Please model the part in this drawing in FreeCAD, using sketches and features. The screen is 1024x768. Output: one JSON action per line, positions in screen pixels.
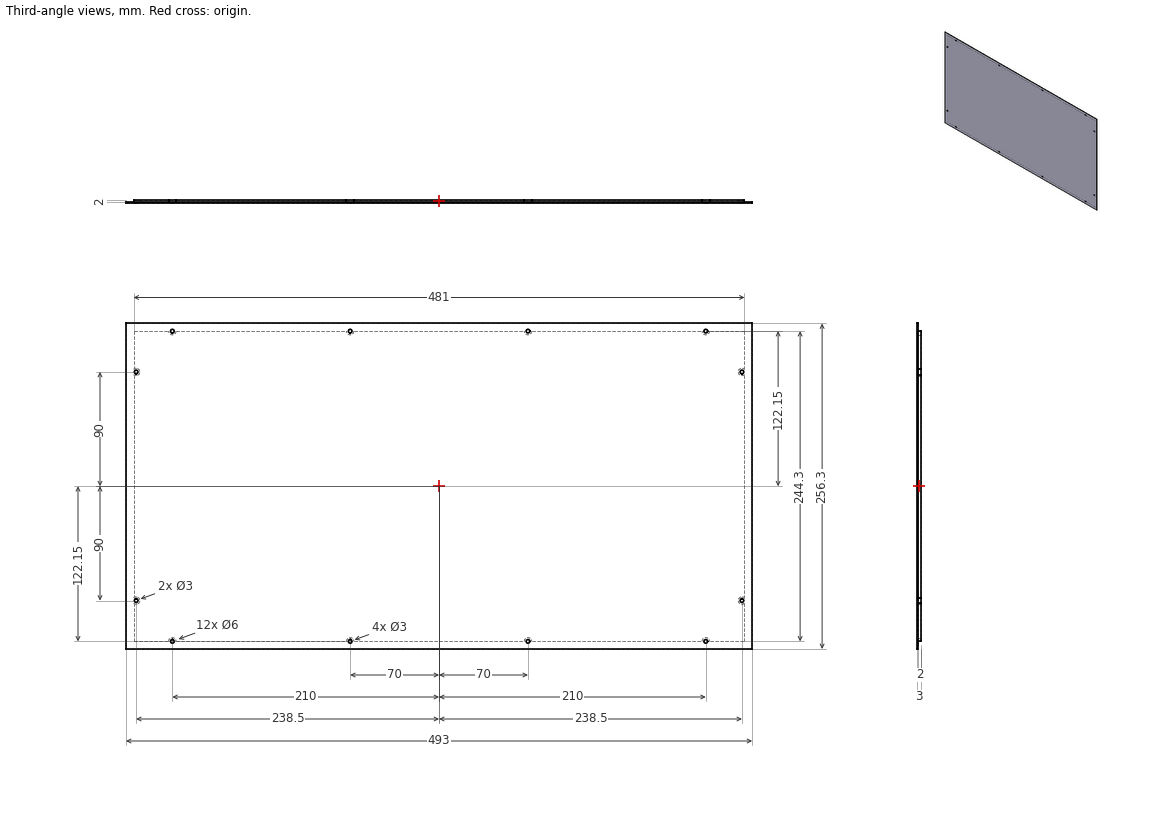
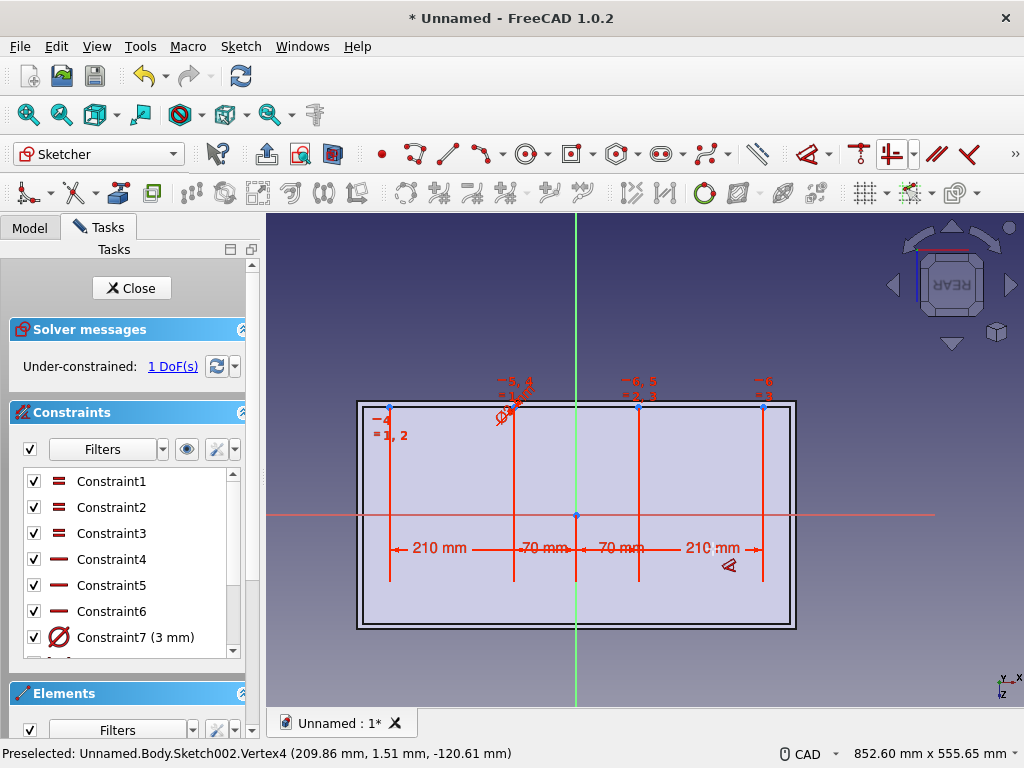
{"action": "left_click", "coordinate": [514, 408]}
{"action": "left_click", "coordinate": [480, 462]}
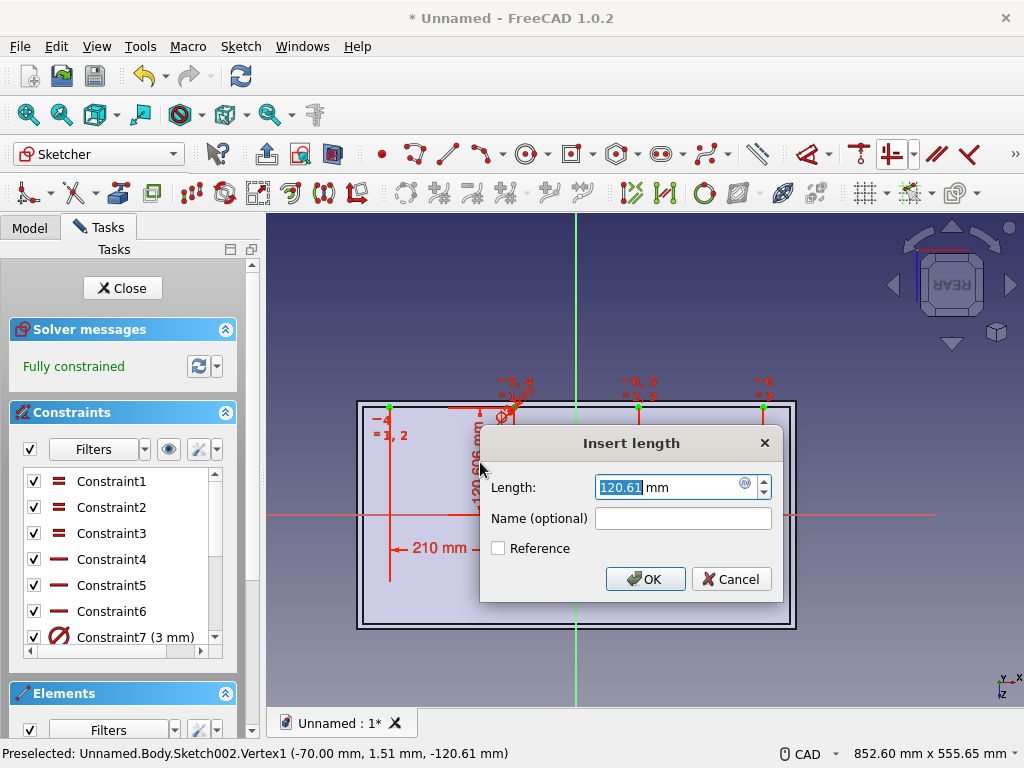
{"action": "type", "text": "122.15"}
{"action": "key", "text": "Return"}
{"action": "key", "text": "Escape"}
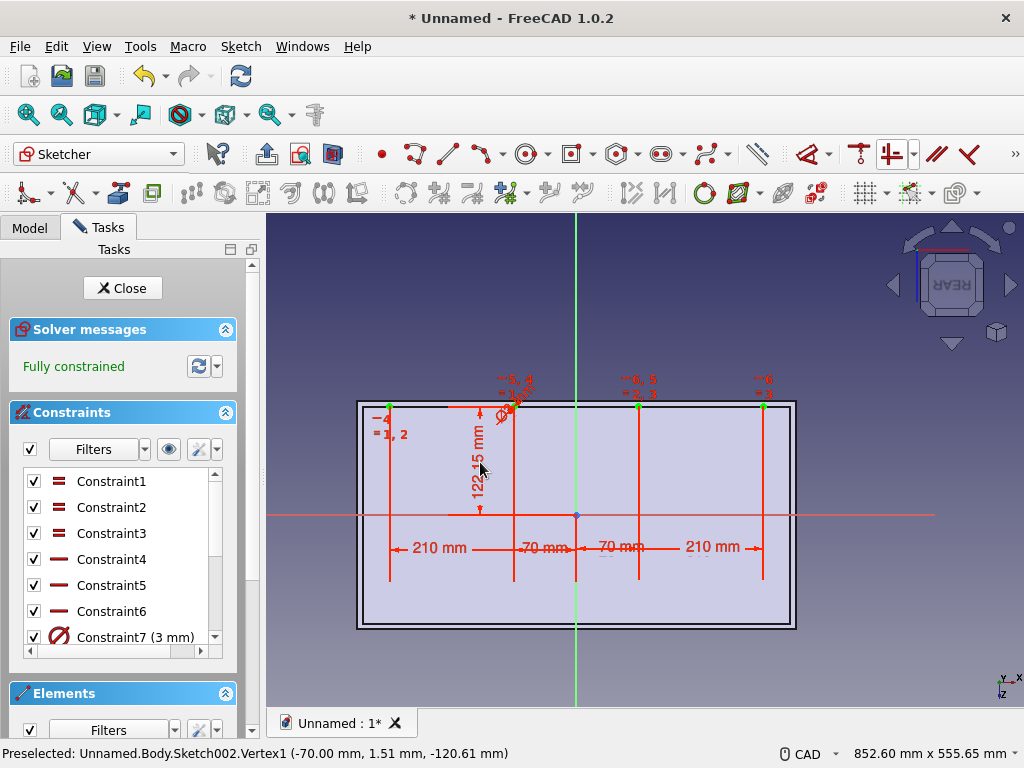
{"action": "left_click", "coordinate": [123, 288]}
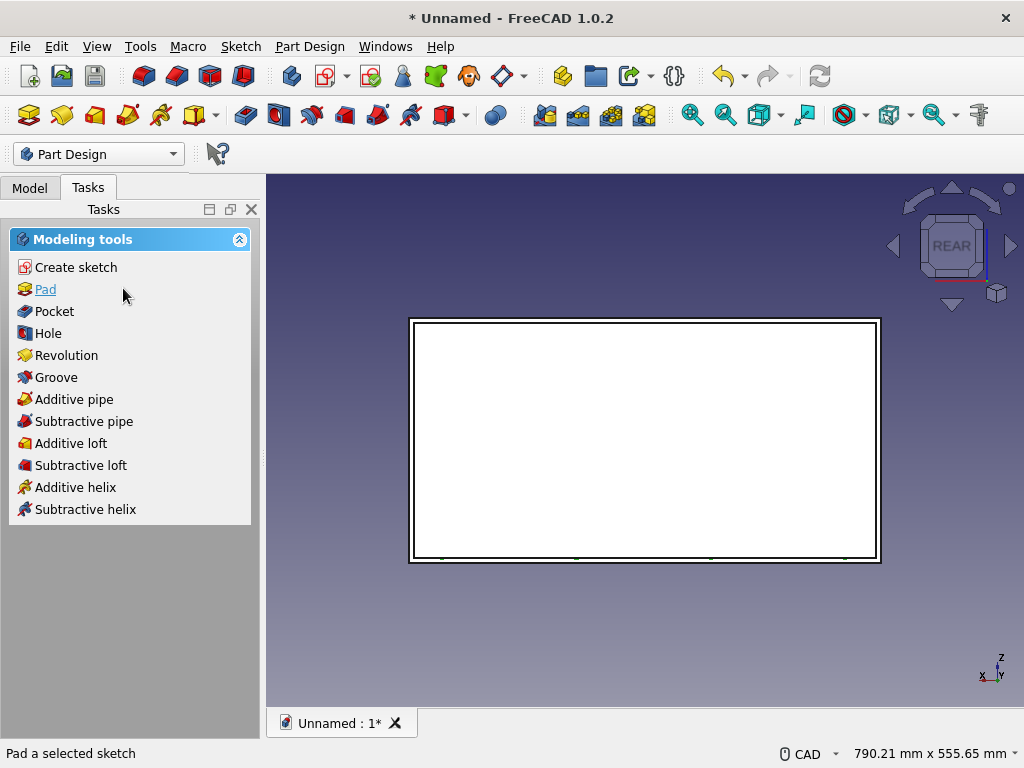
{"action": "left_click", "coordinate": [246, 116]}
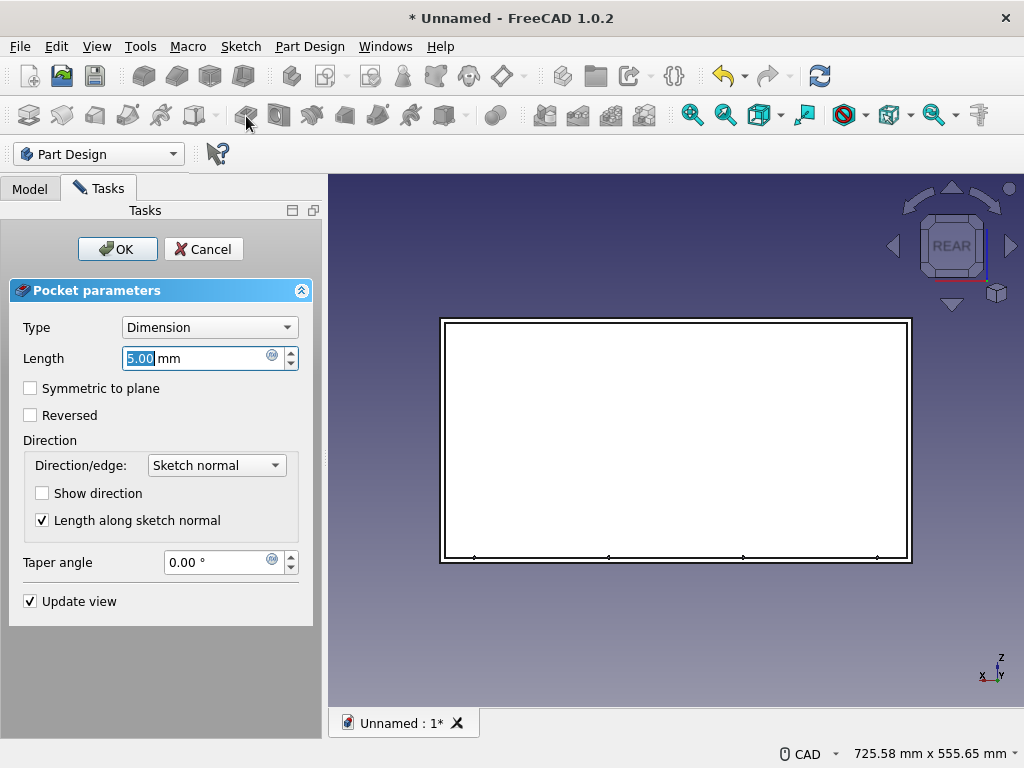
{"action": "left_click", "coordinate": [210, 328]}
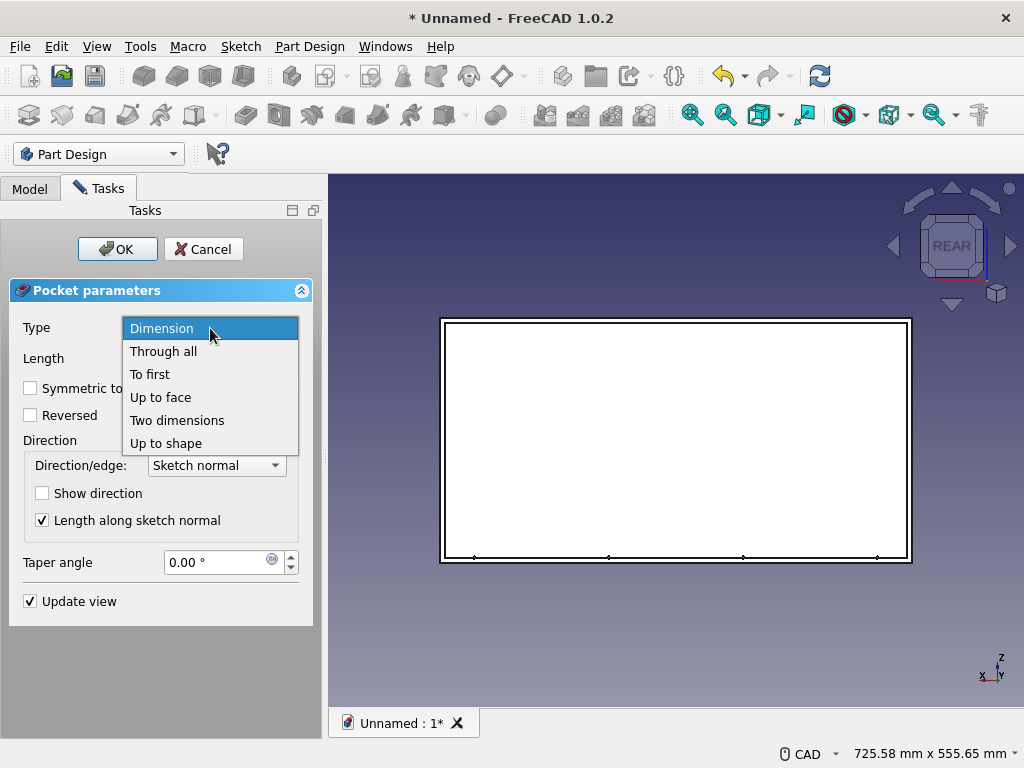
{"action": "left_click", "coordinate": [208, 352]}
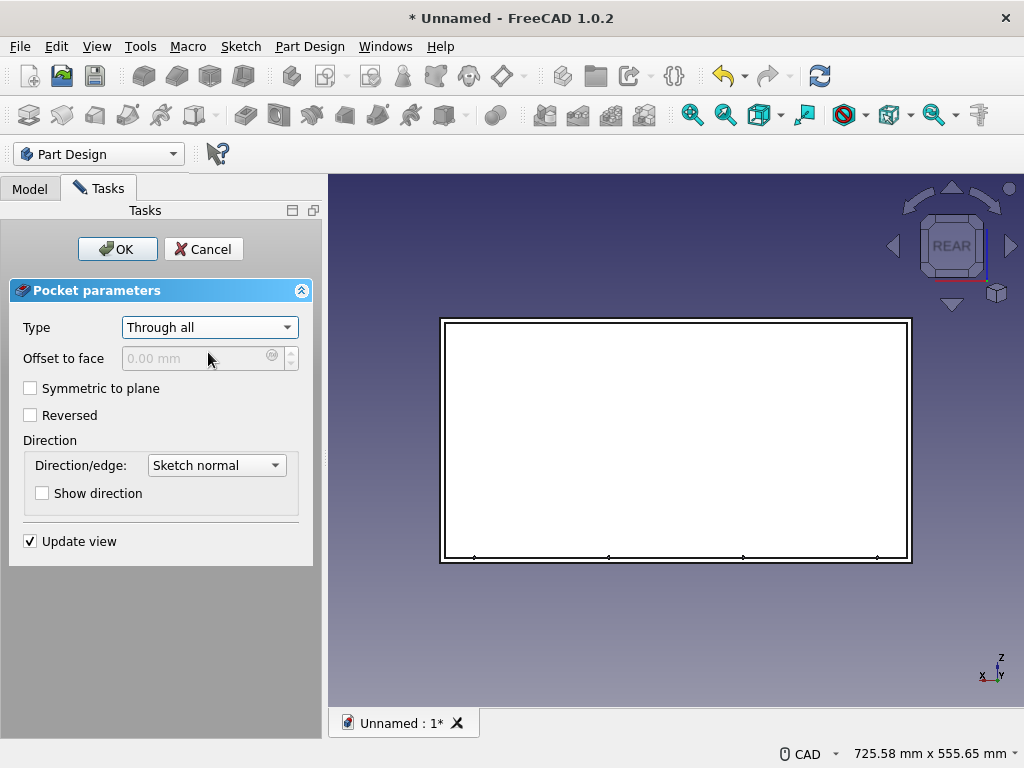
{"action": "left_click", "coordinate": [118, 249]}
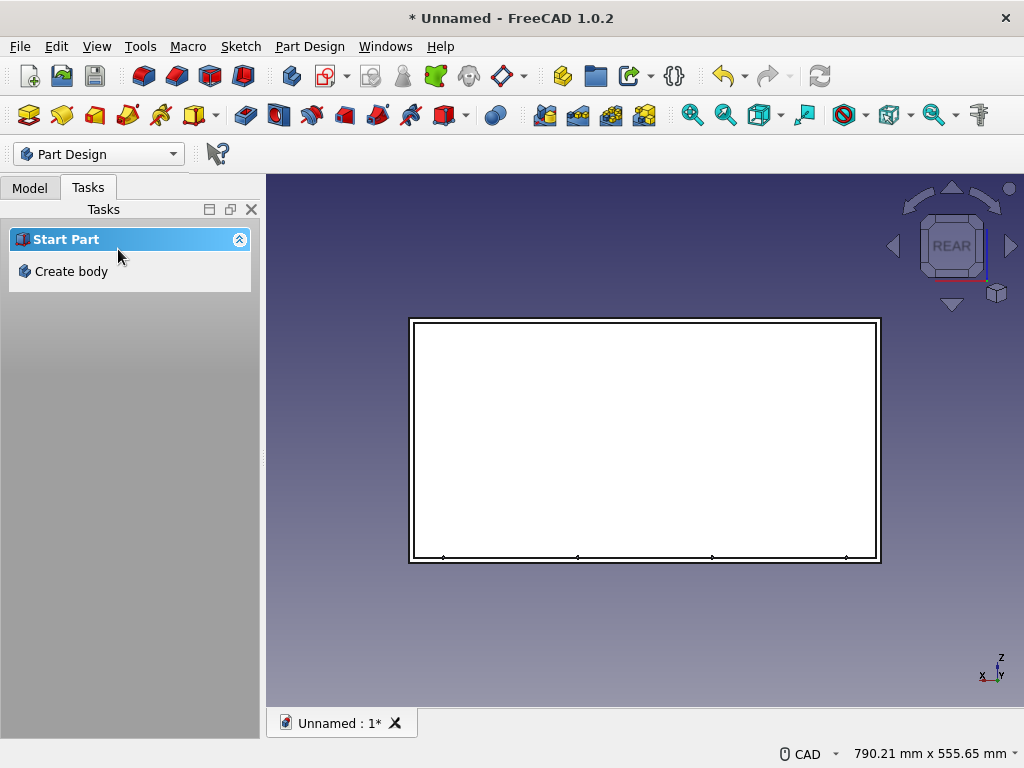
{"action": "left_click", "coordinate": [30, 188]}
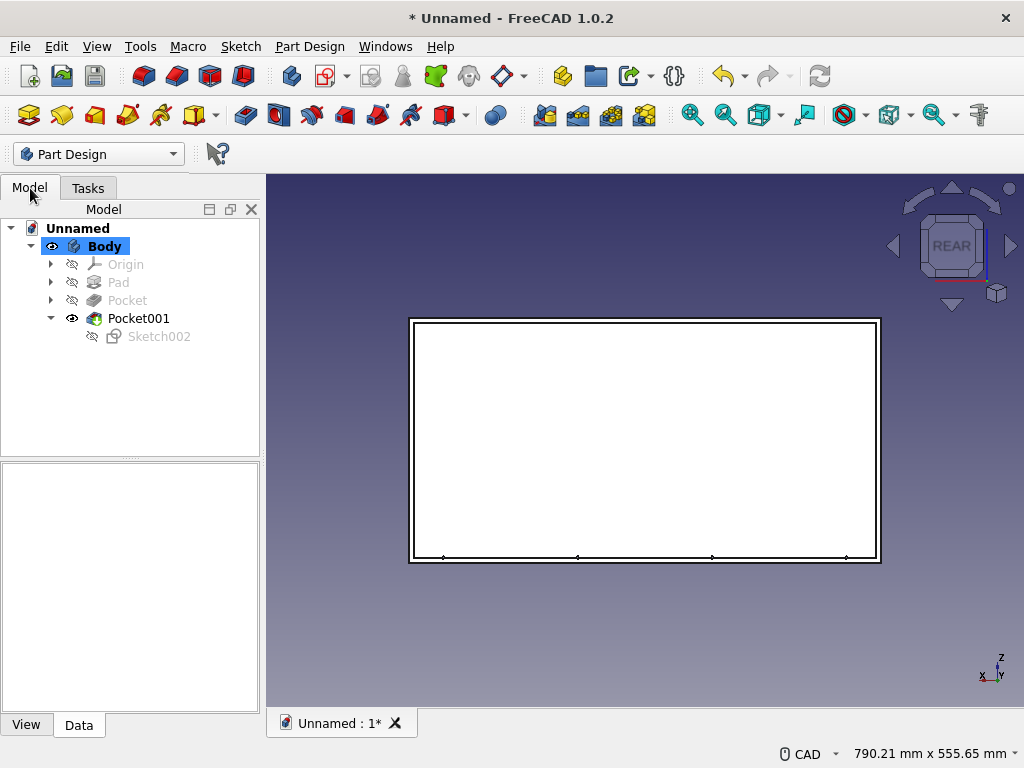
{"action": "left_click", "coordinate": [117, 318]}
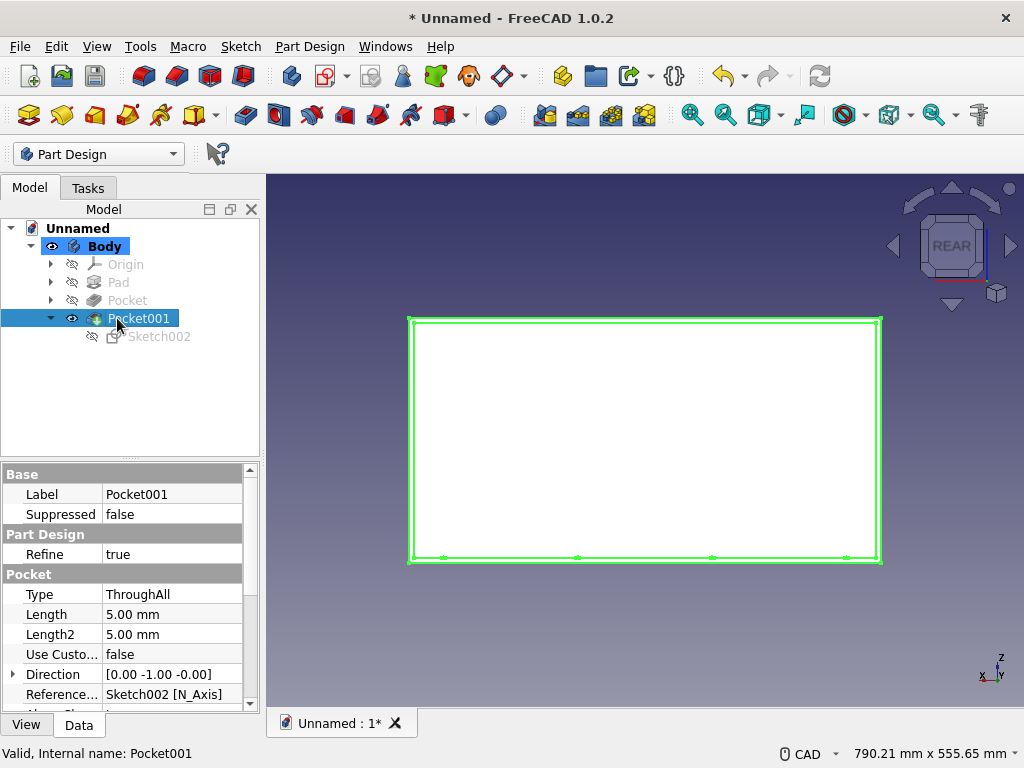
{"action": "left_click", "coordinate": [545, 116]}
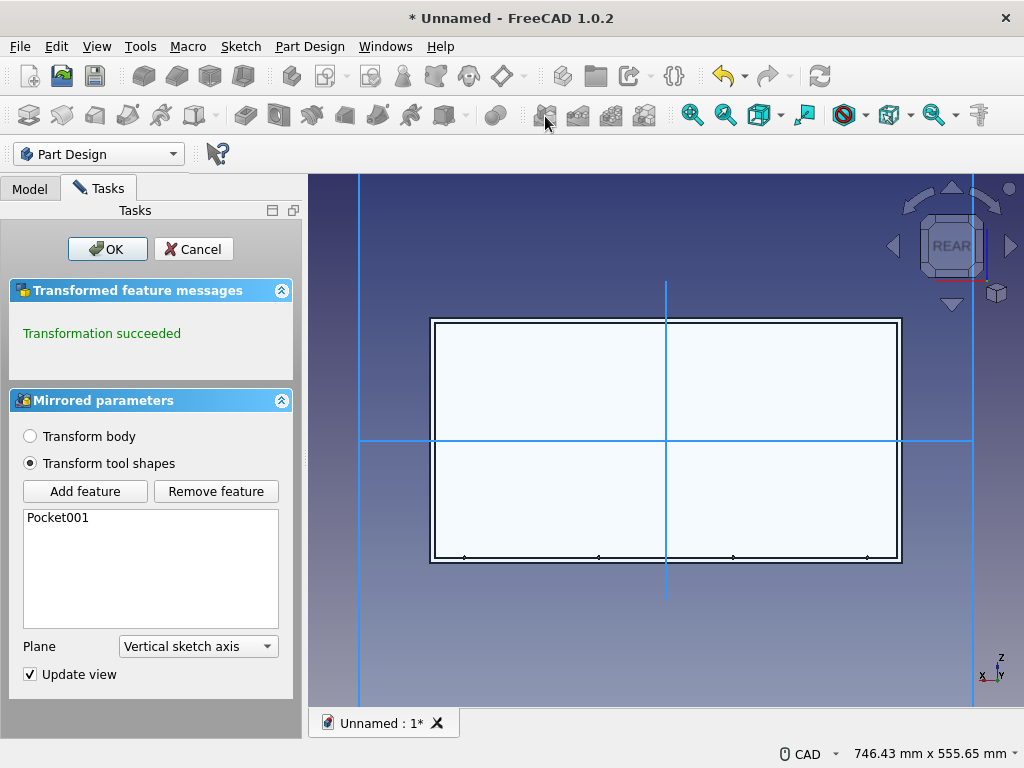
{"action": "left_click", "coordinate": [199, 646]}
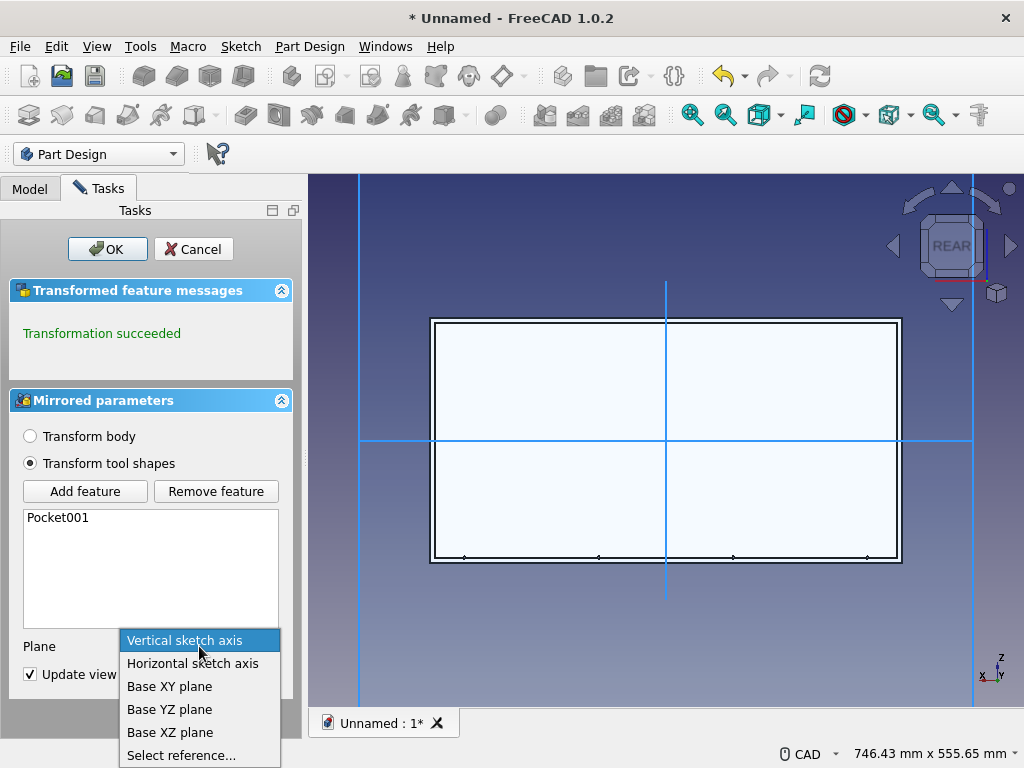
{"action": "left_click", "coordinate": [198, 686]}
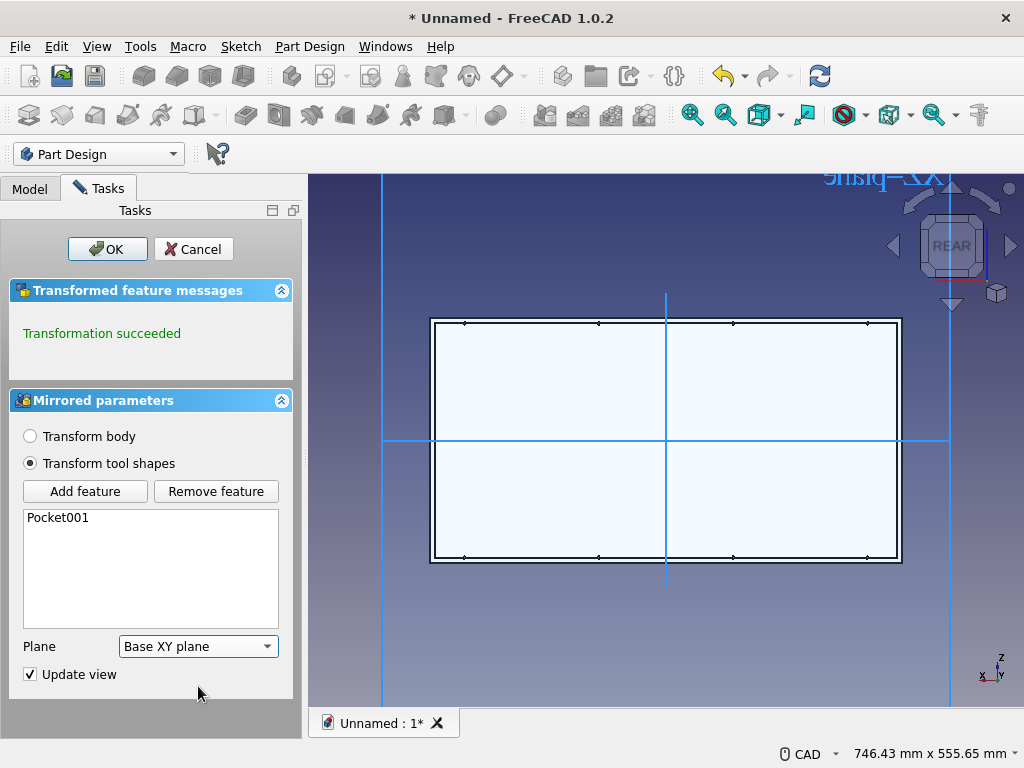
{"action": "left_click", "coordinate": [108, 249]}